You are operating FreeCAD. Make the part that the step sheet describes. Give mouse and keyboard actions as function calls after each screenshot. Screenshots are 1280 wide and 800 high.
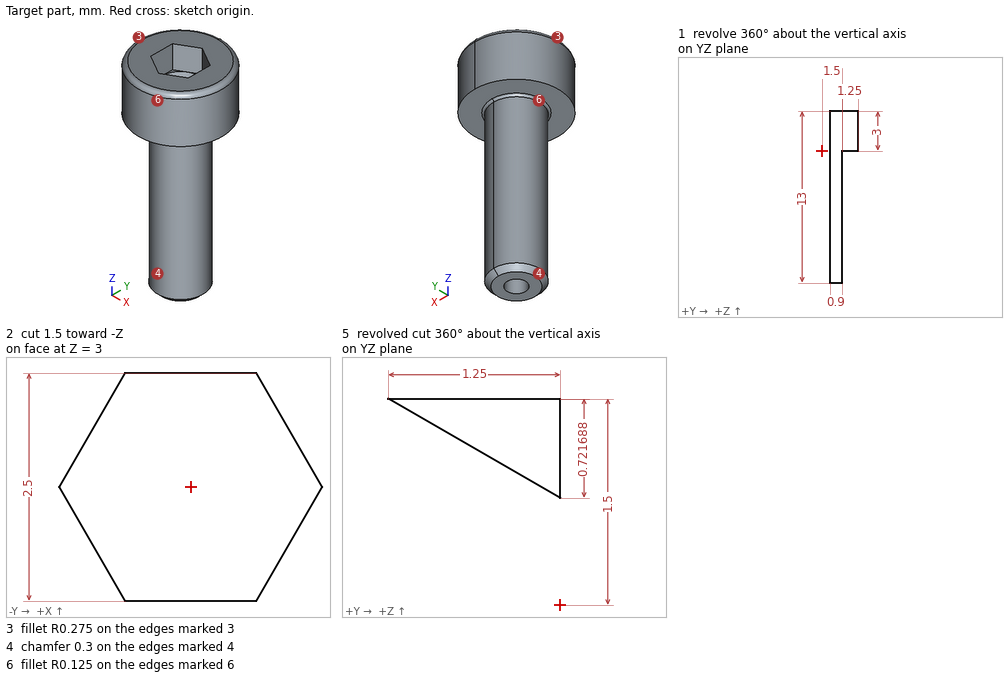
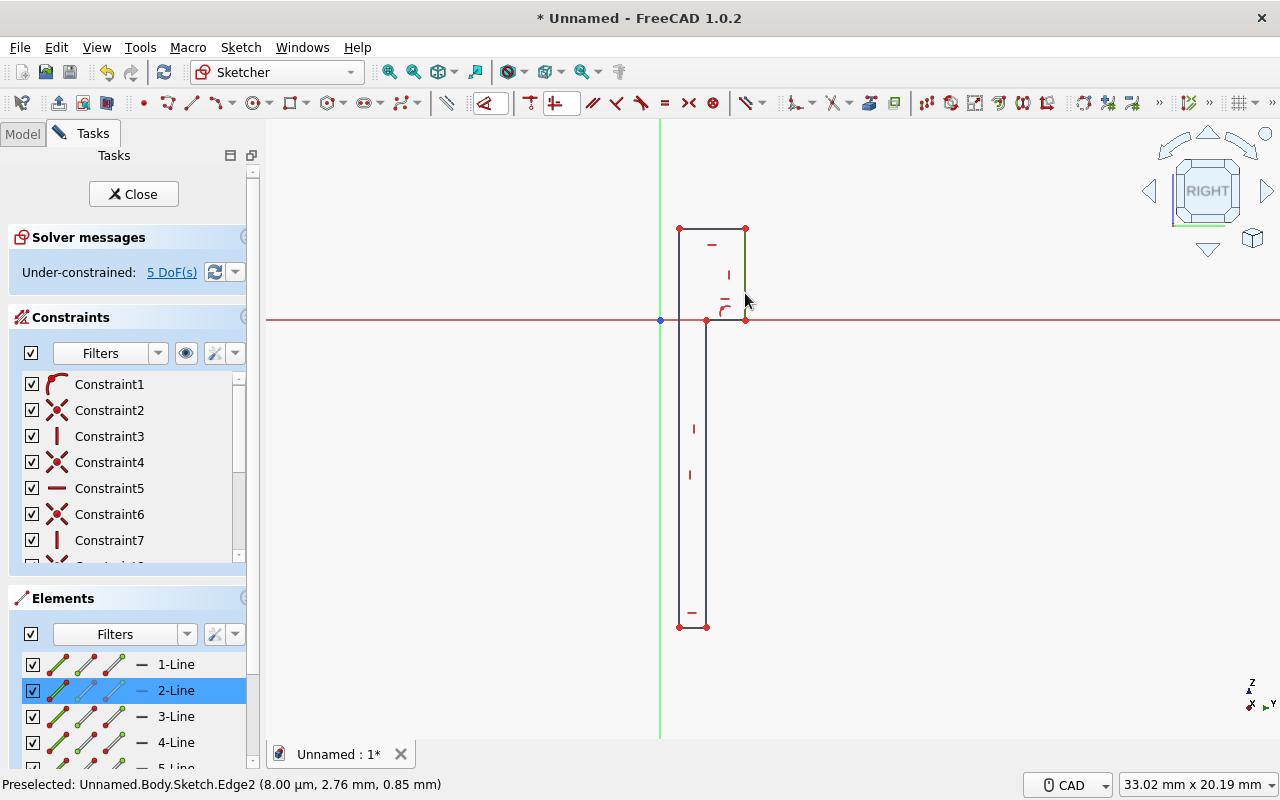
click(502, 104)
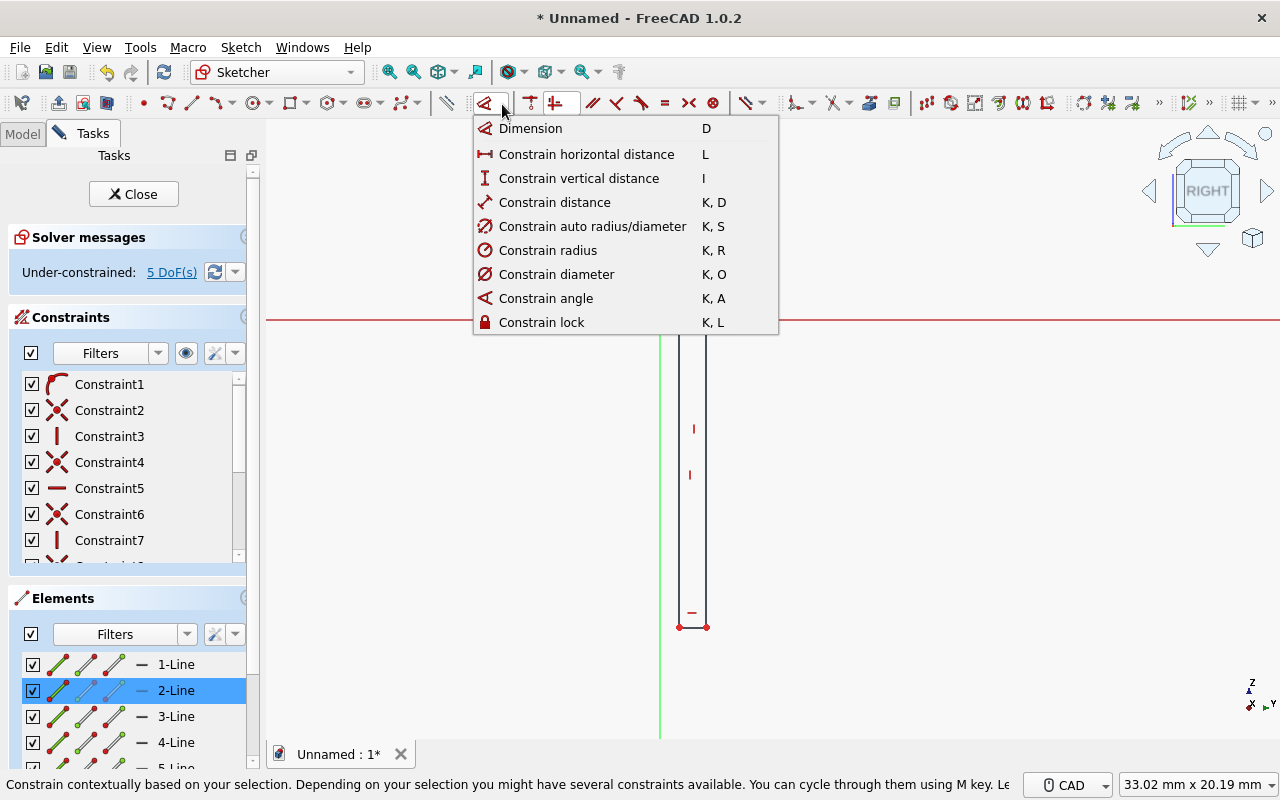
click(626, 178)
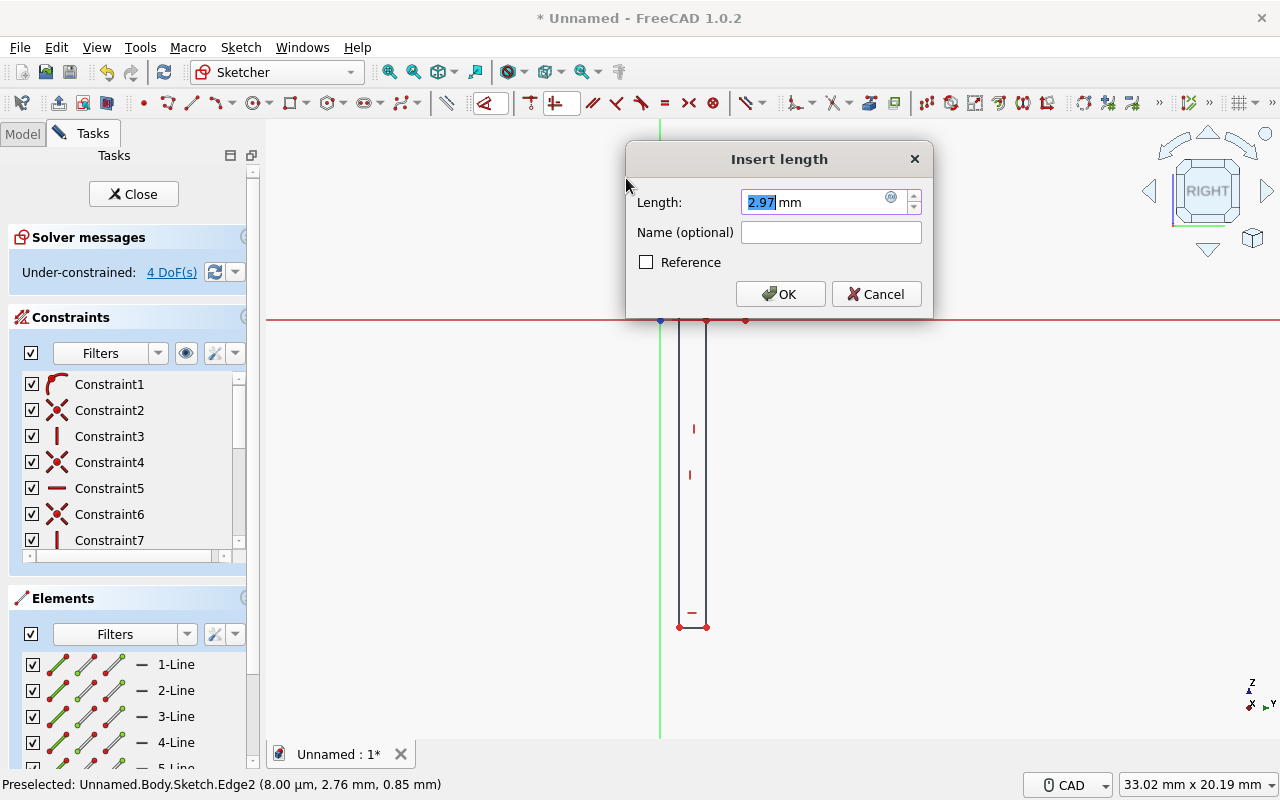
text(3)
key(Return)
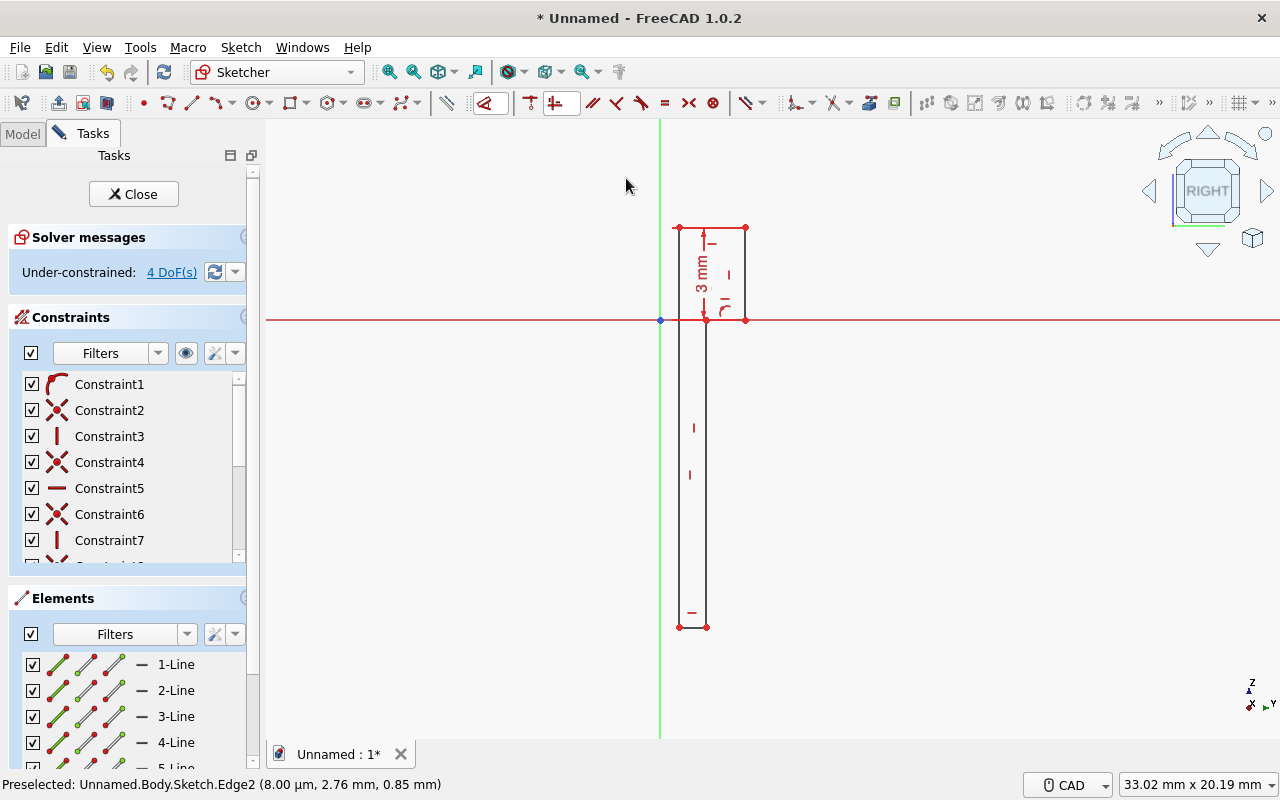
click(679, 348)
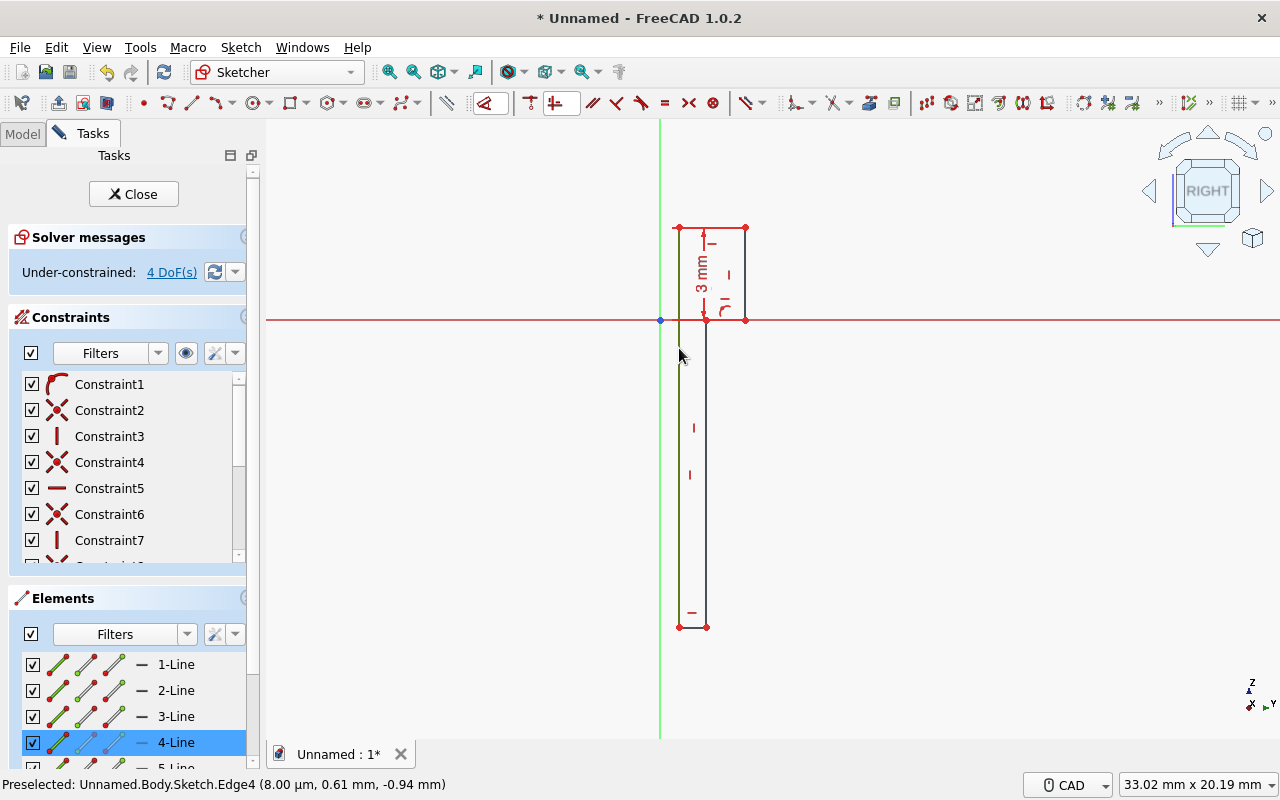
click(502, 104)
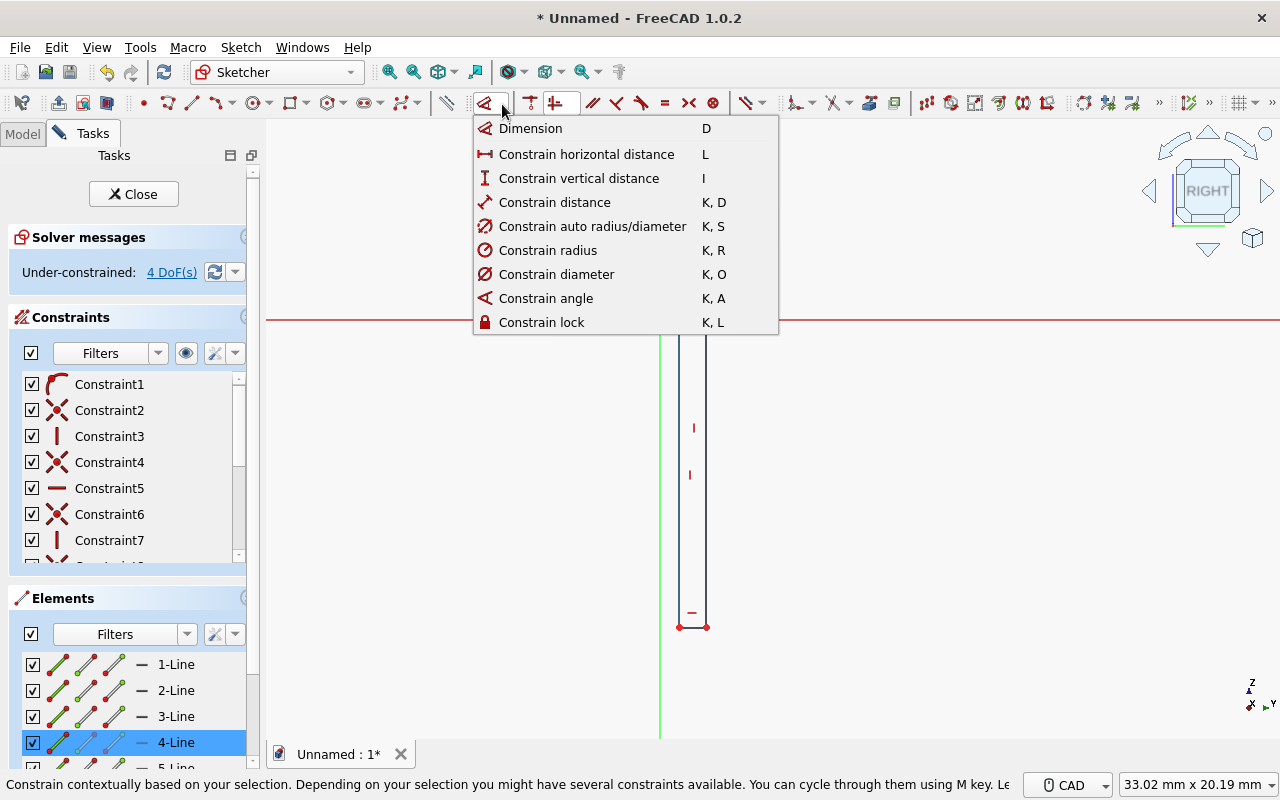
click(626, 178)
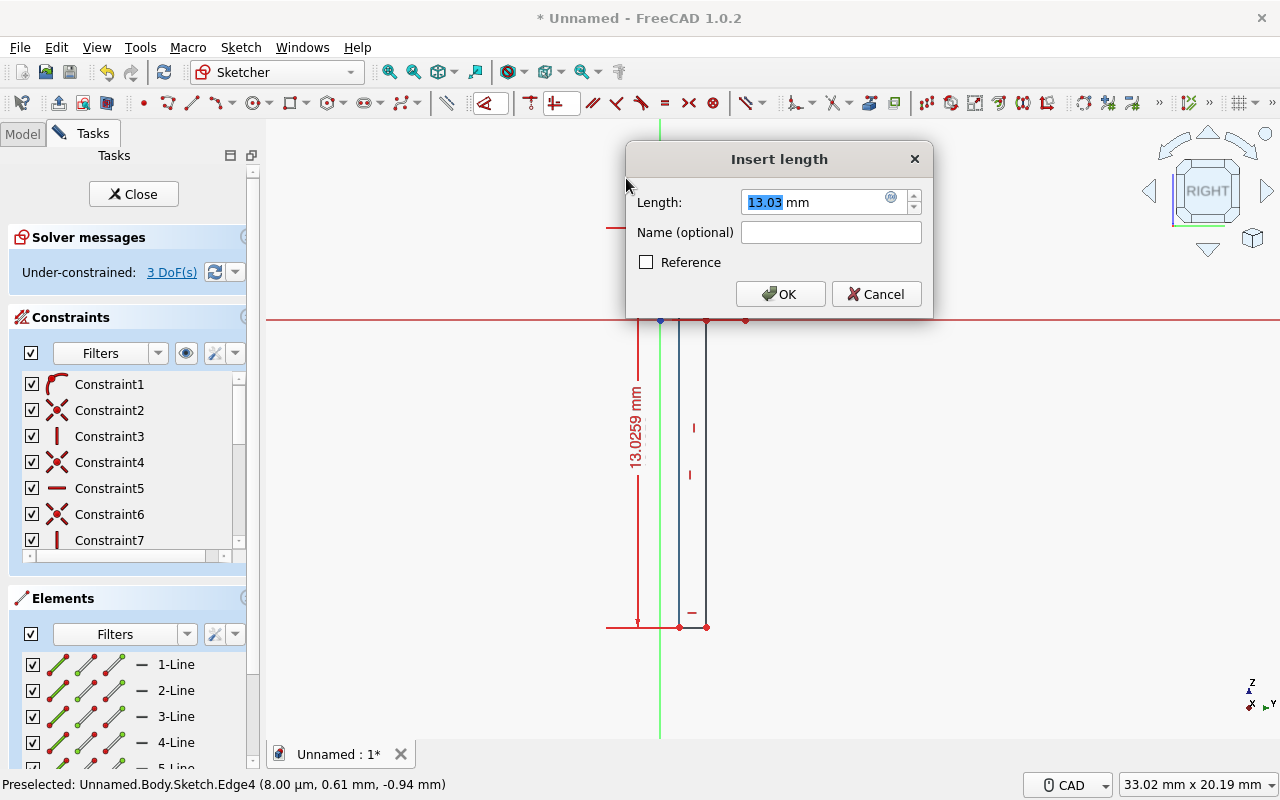
text(13)
key(Return)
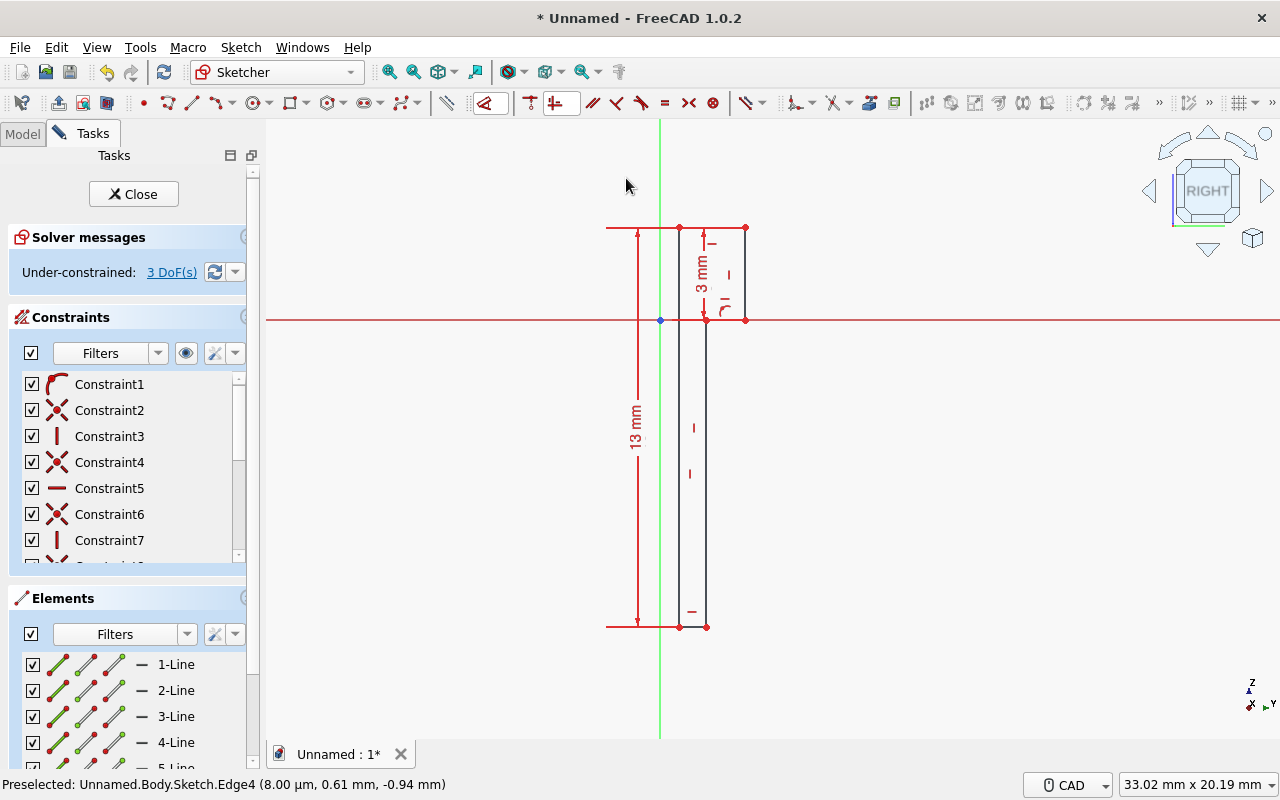
scroll(690, 627, up, 2)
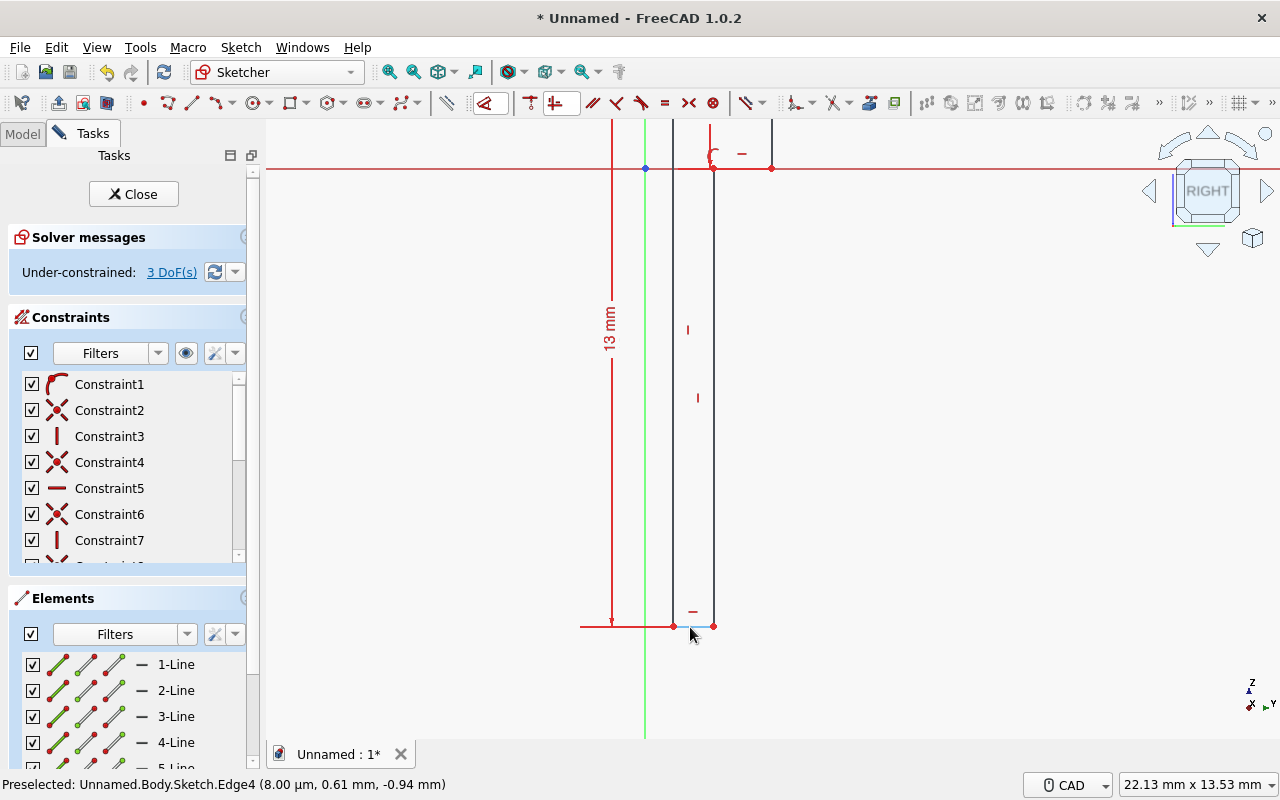
click(689, 627)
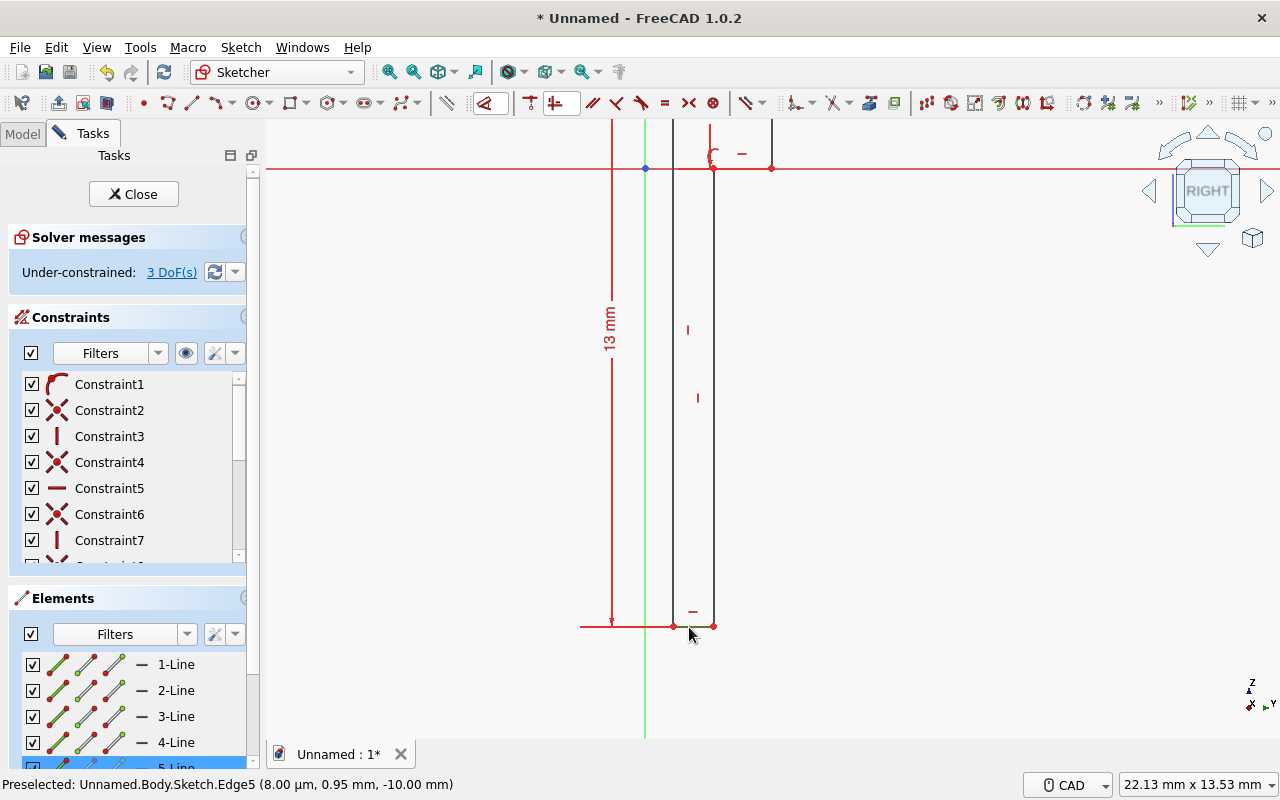
key(l)